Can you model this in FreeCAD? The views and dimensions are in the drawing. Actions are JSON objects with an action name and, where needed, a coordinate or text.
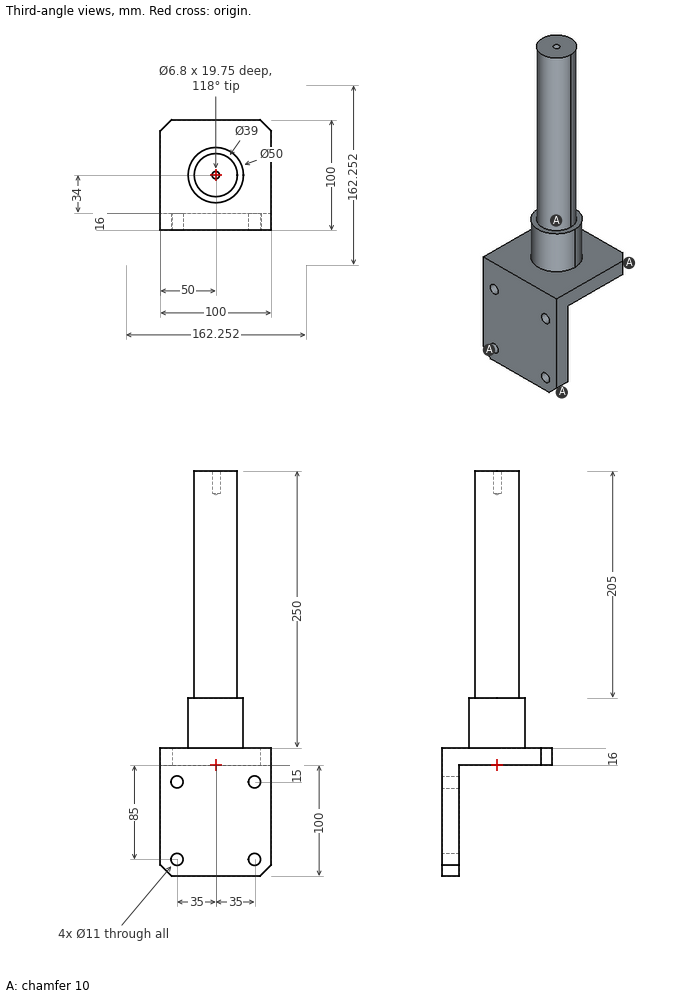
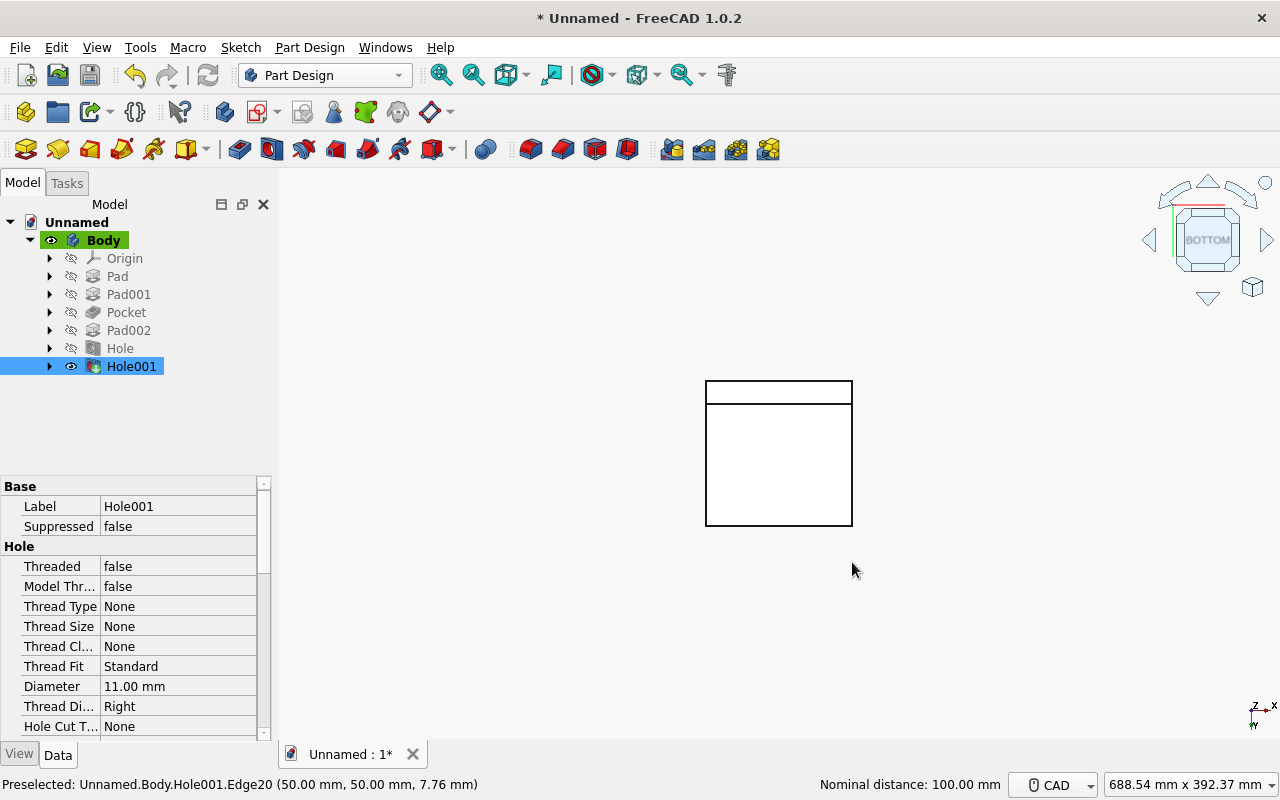
{"action": "left_click", "coordinate": [706, 391], "text": "ctrl"}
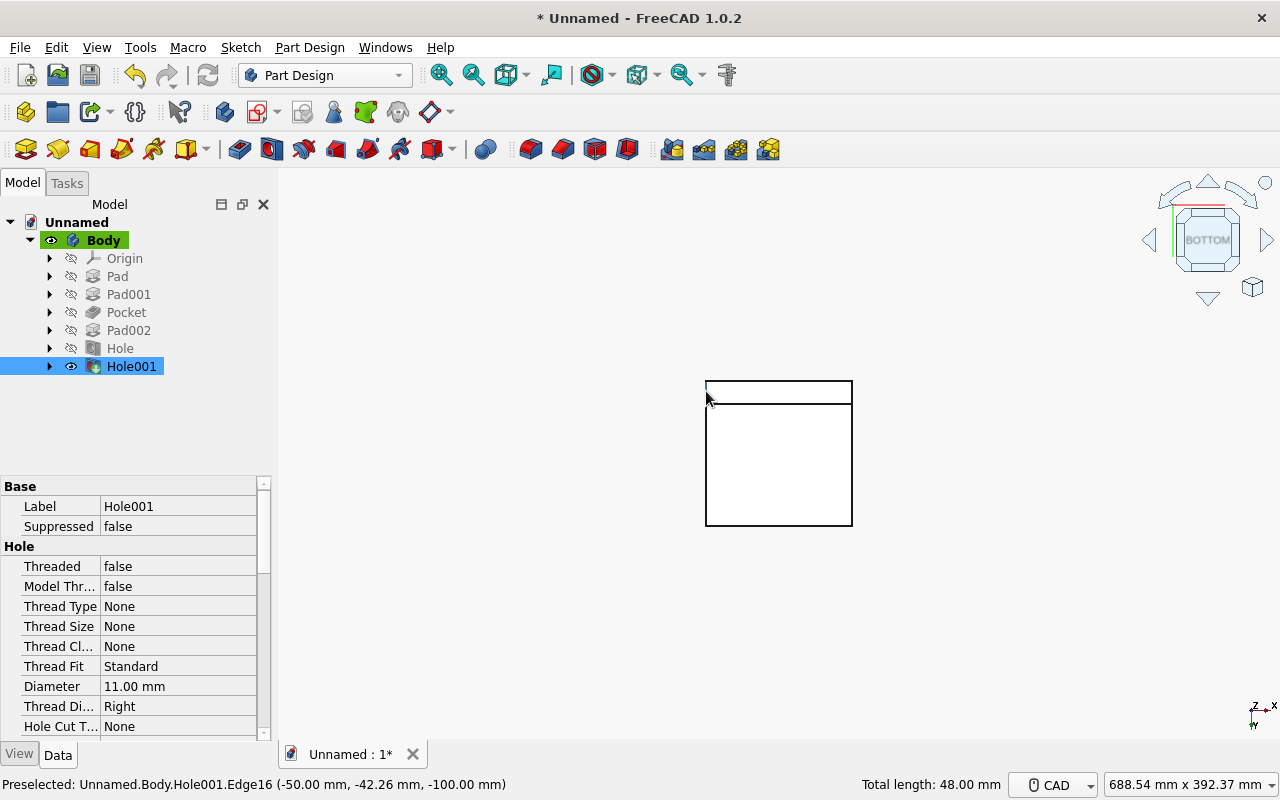
{"action": "left_click", "coordinate": [852, 391], "text": "ctrl"}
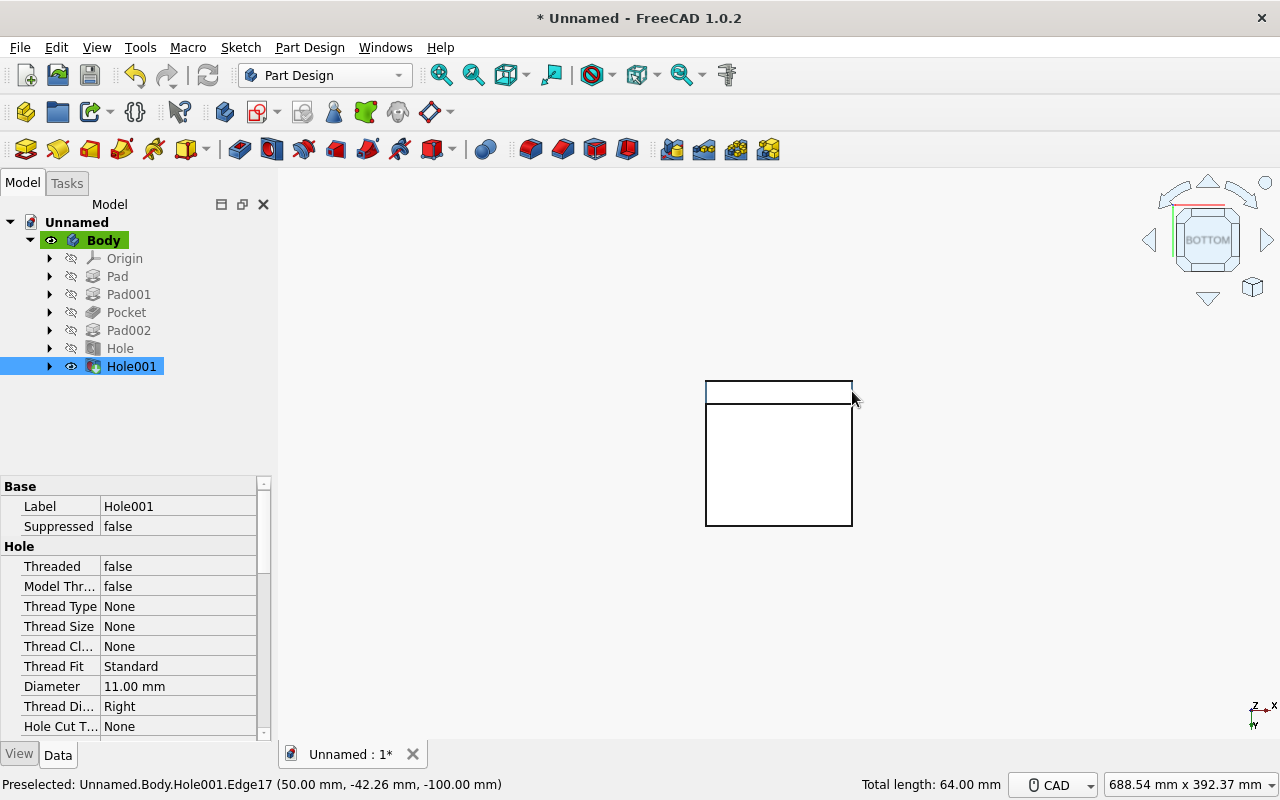
{"action": "left_click", "coordinate": [564, 150]}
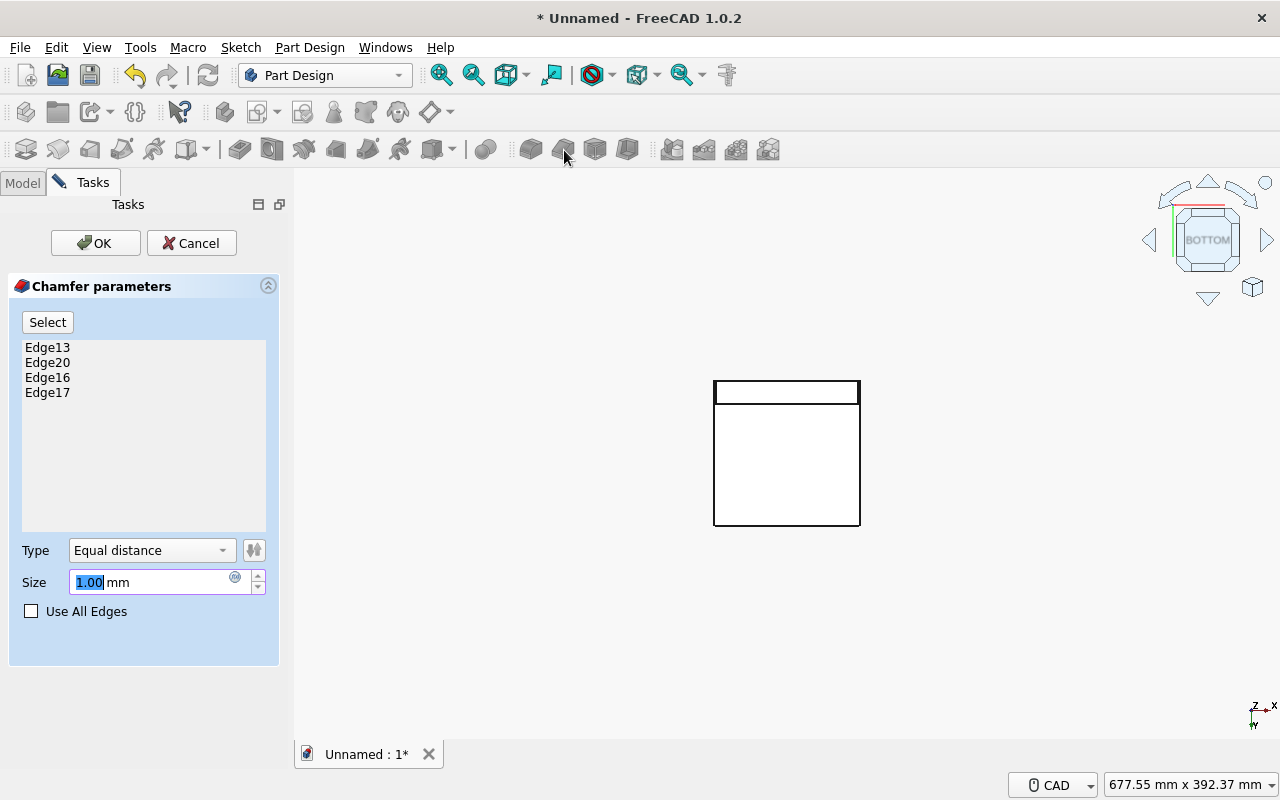
{"action": "type", "text": "10"}
{"action": "key", "text": "Tab"}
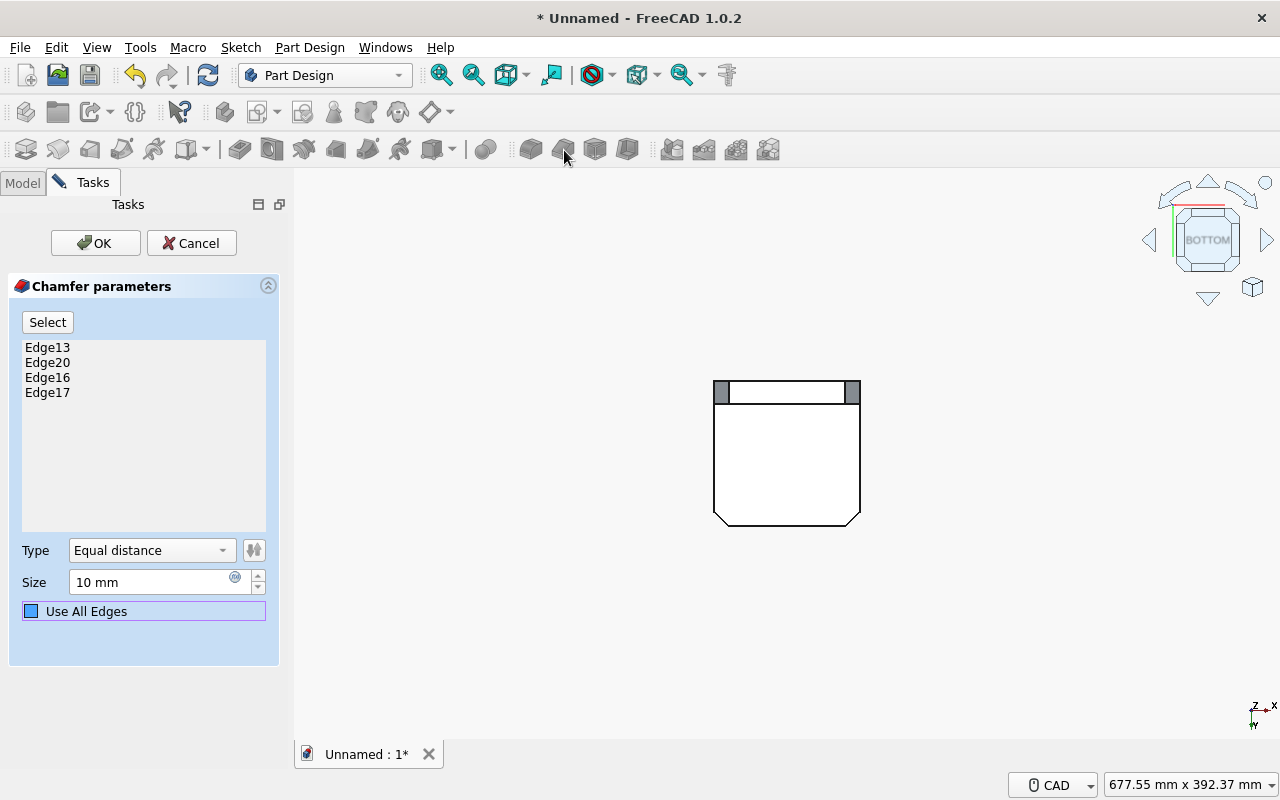
{"action": "left_click", "coordinate": [96, 243]}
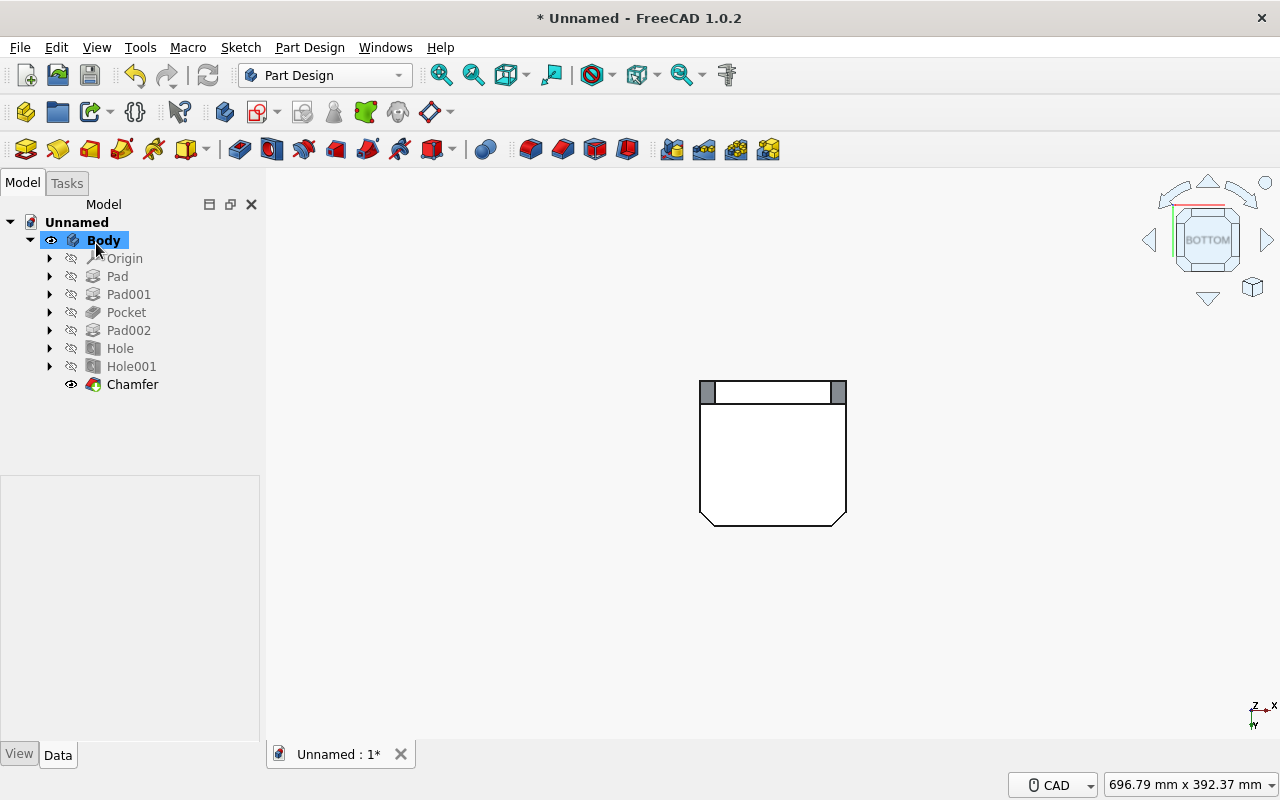
{"action": "key", "text": "0"}